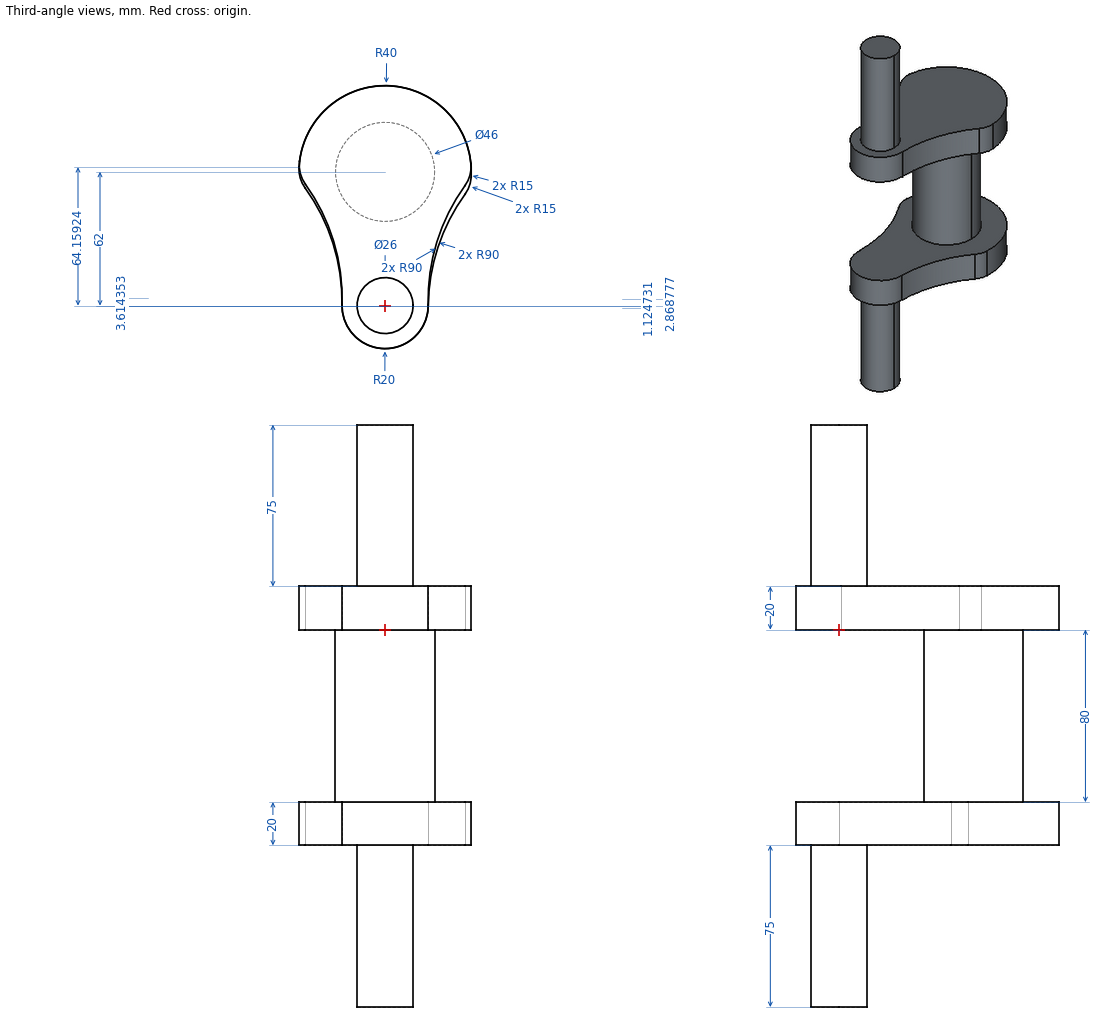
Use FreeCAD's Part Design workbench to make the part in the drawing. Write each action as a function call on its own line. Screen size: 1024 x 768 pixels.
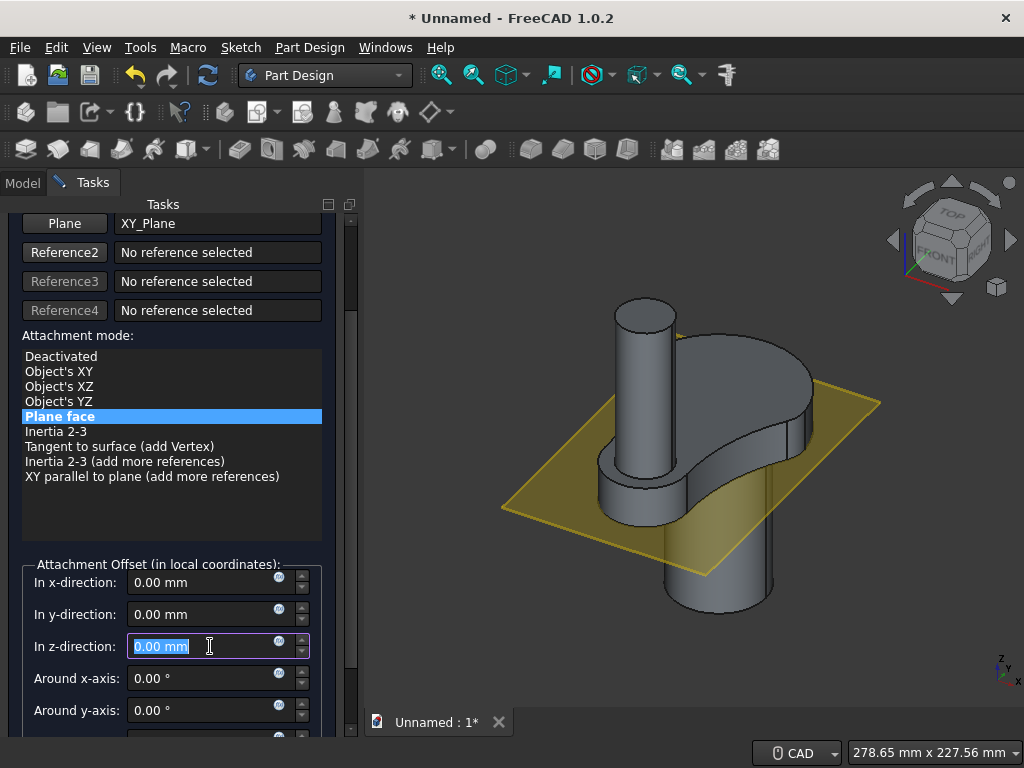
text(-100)
key(Tab)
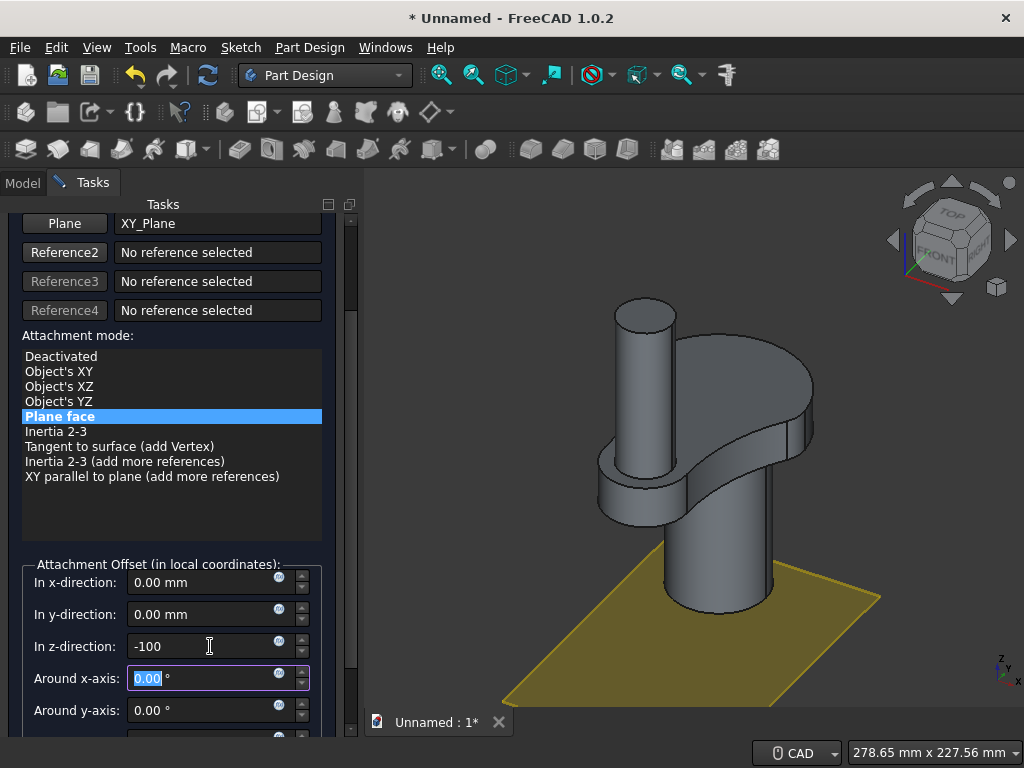
scroll(351, 475, up, 3)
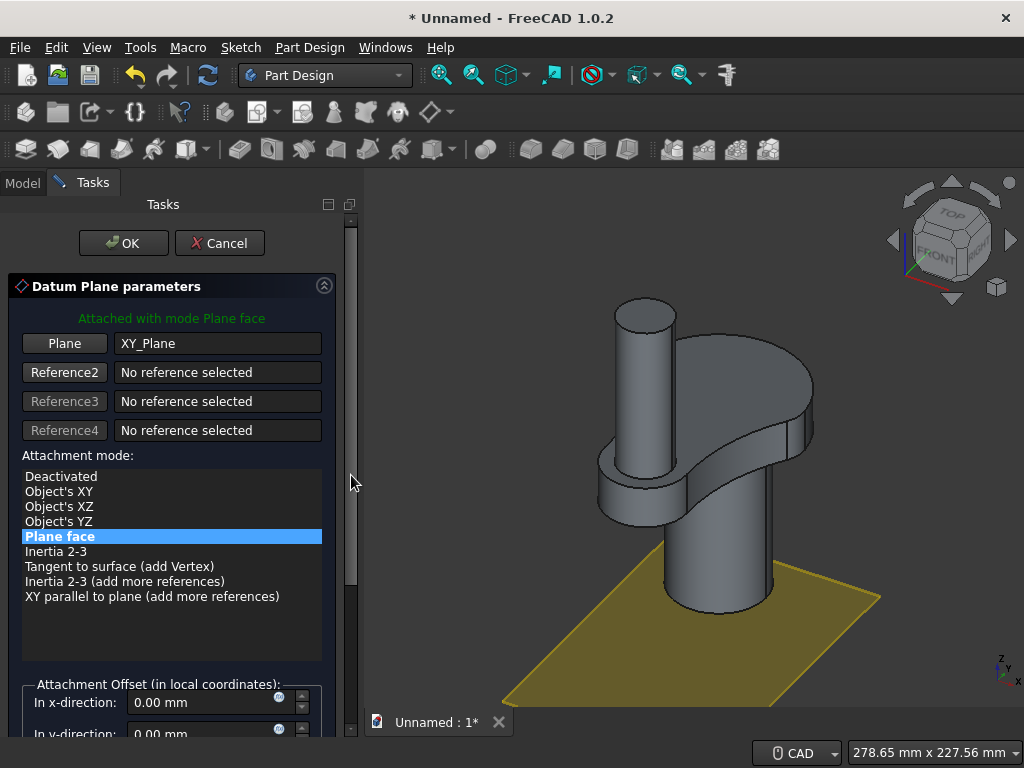
click(124, 243)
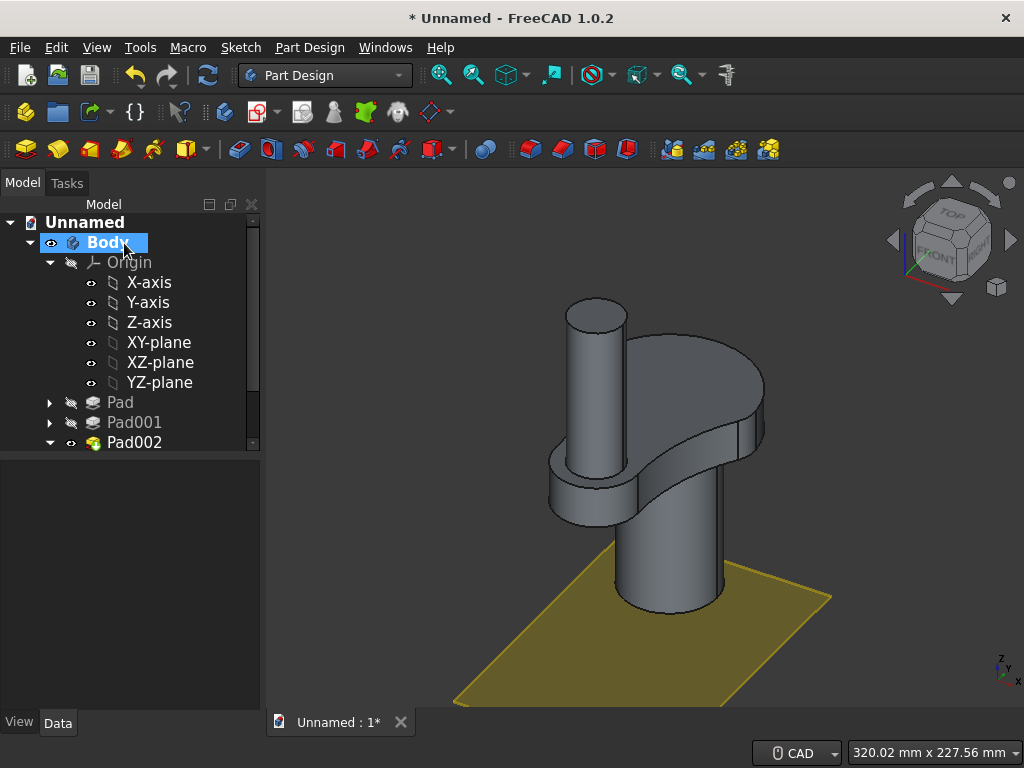
scroll(100, 338, down, 3)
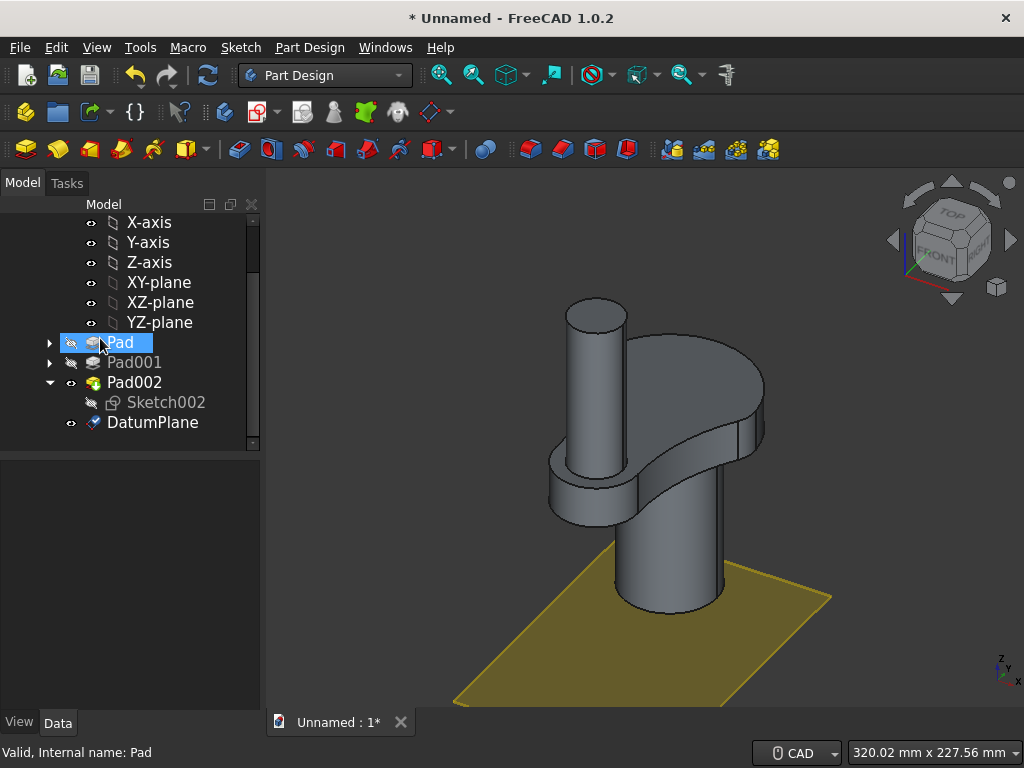
click(116, 423)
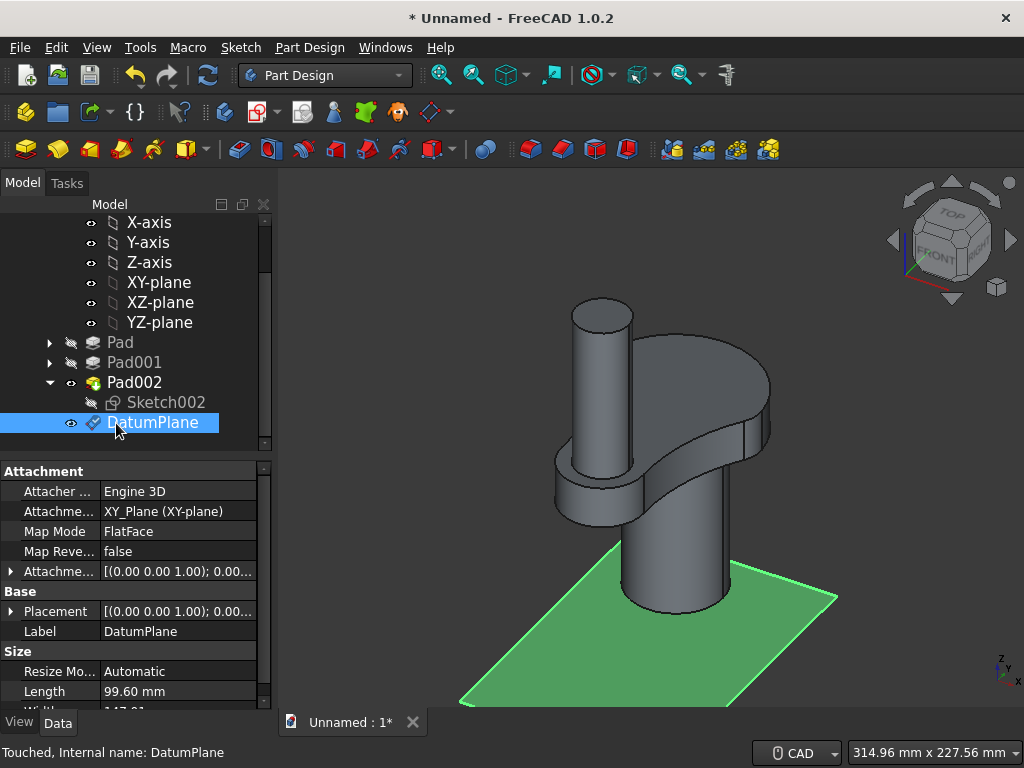
click(258, 112)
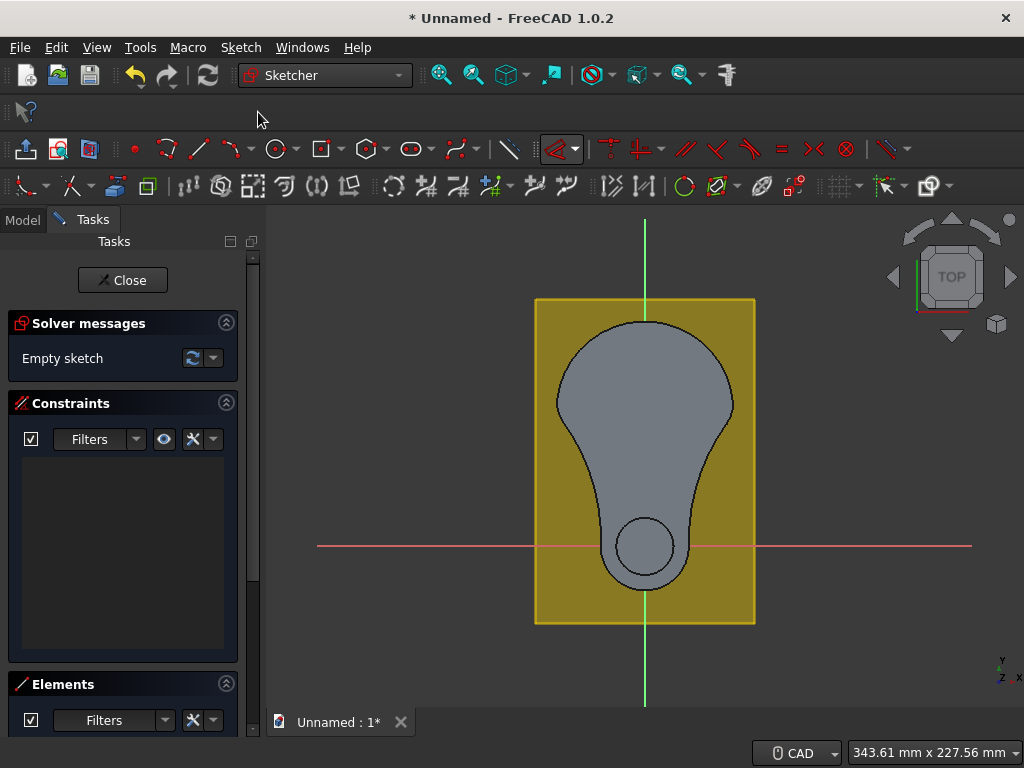
click(90, 150)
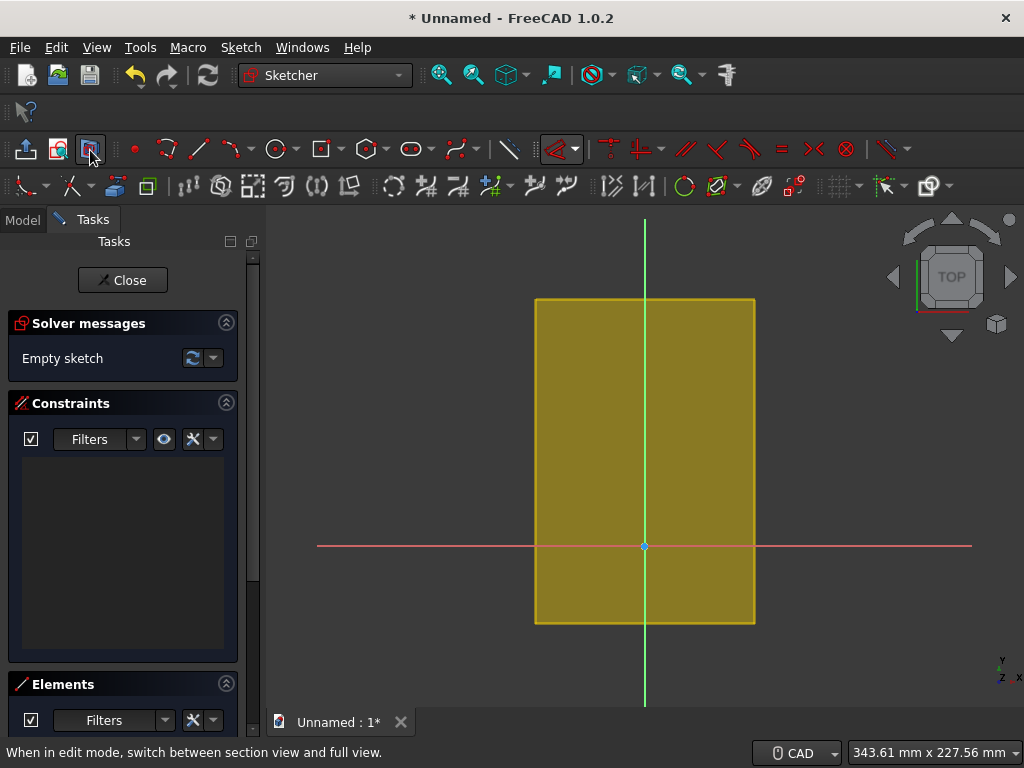
key(g)
key(3)
key(a)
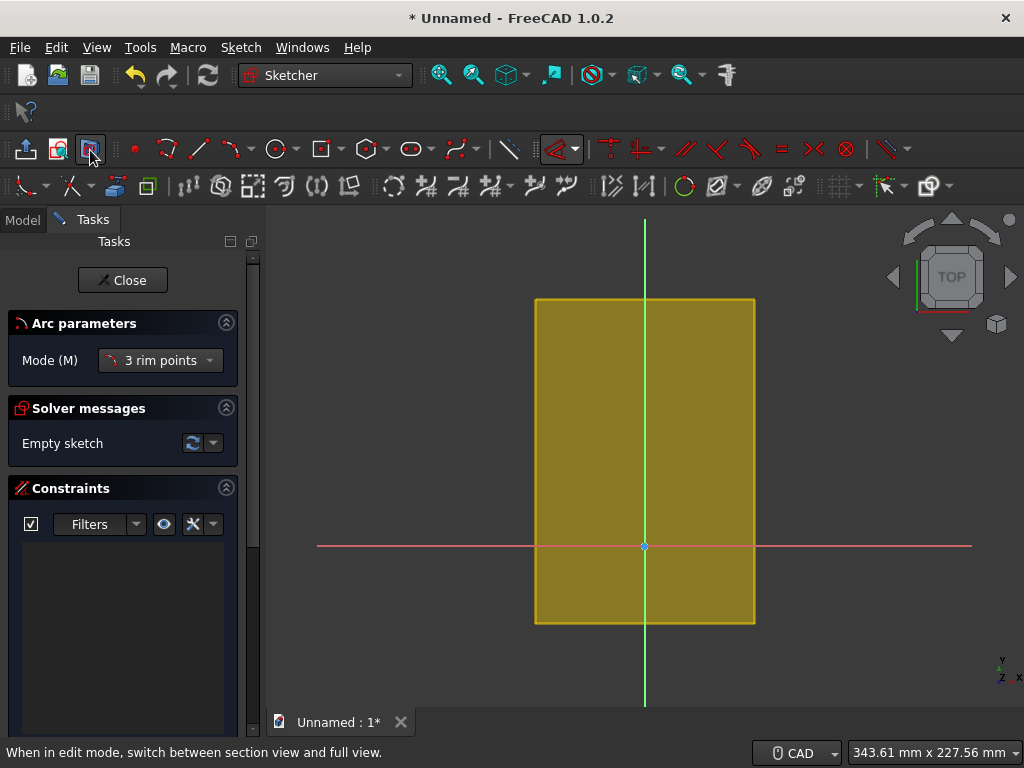
scroll(689, 547, up, 18)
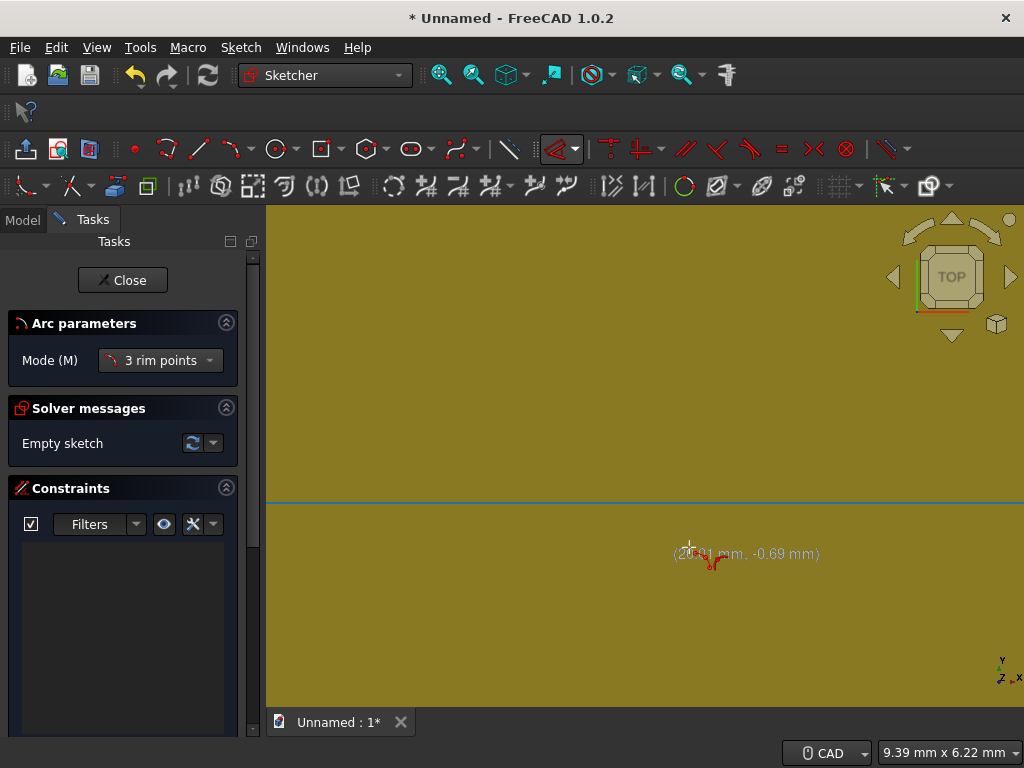
click(669, 520)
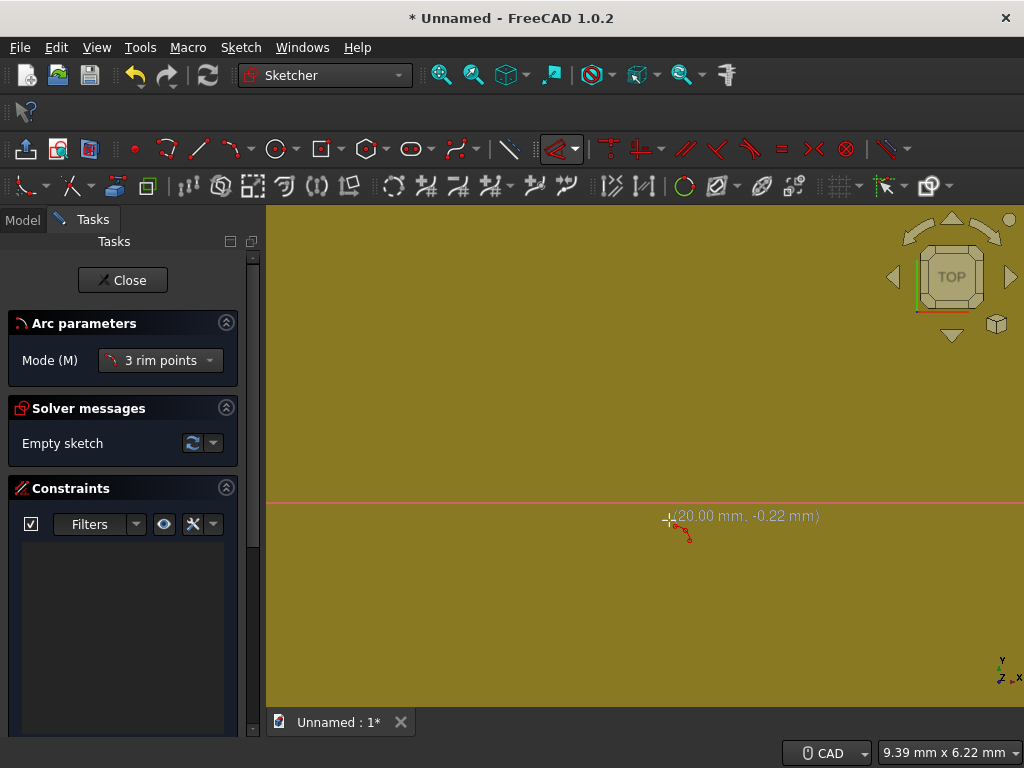
scroll(629, 569, down, 17)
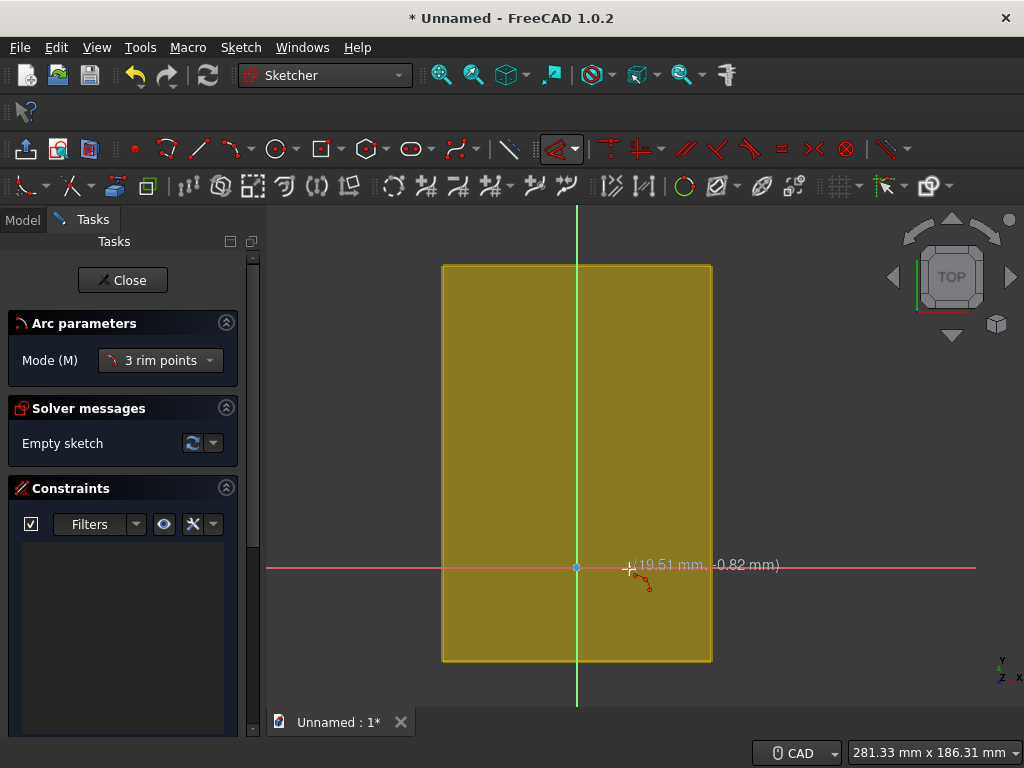
click(677, 428)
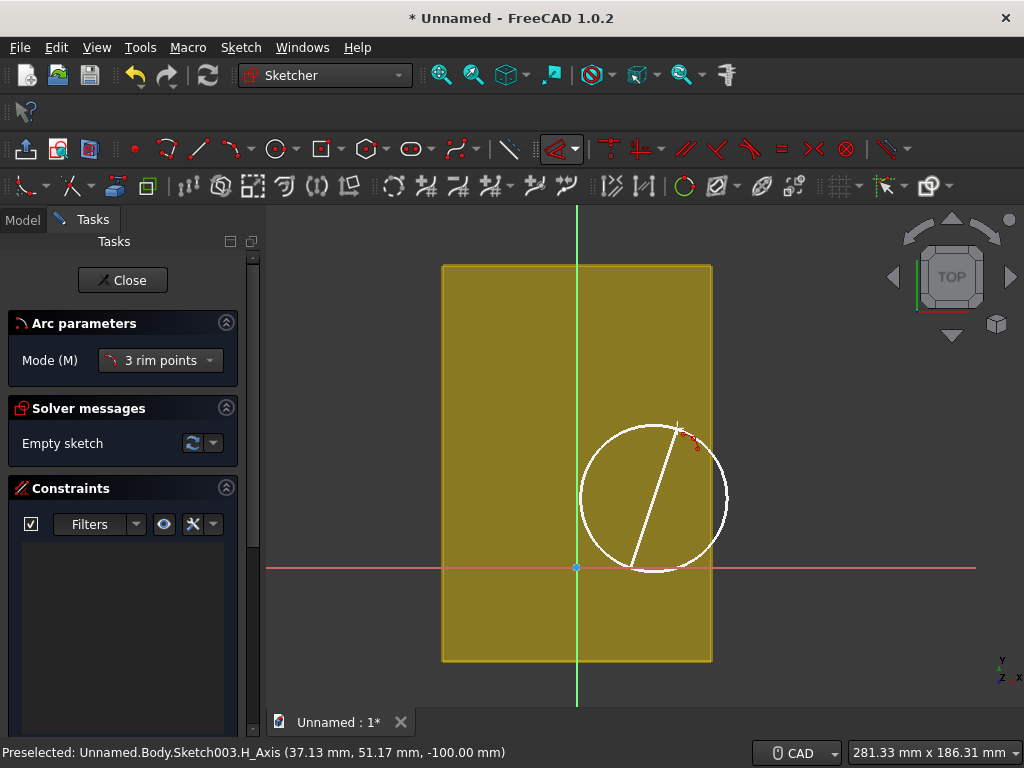
scroll(643, 495, up, 2)